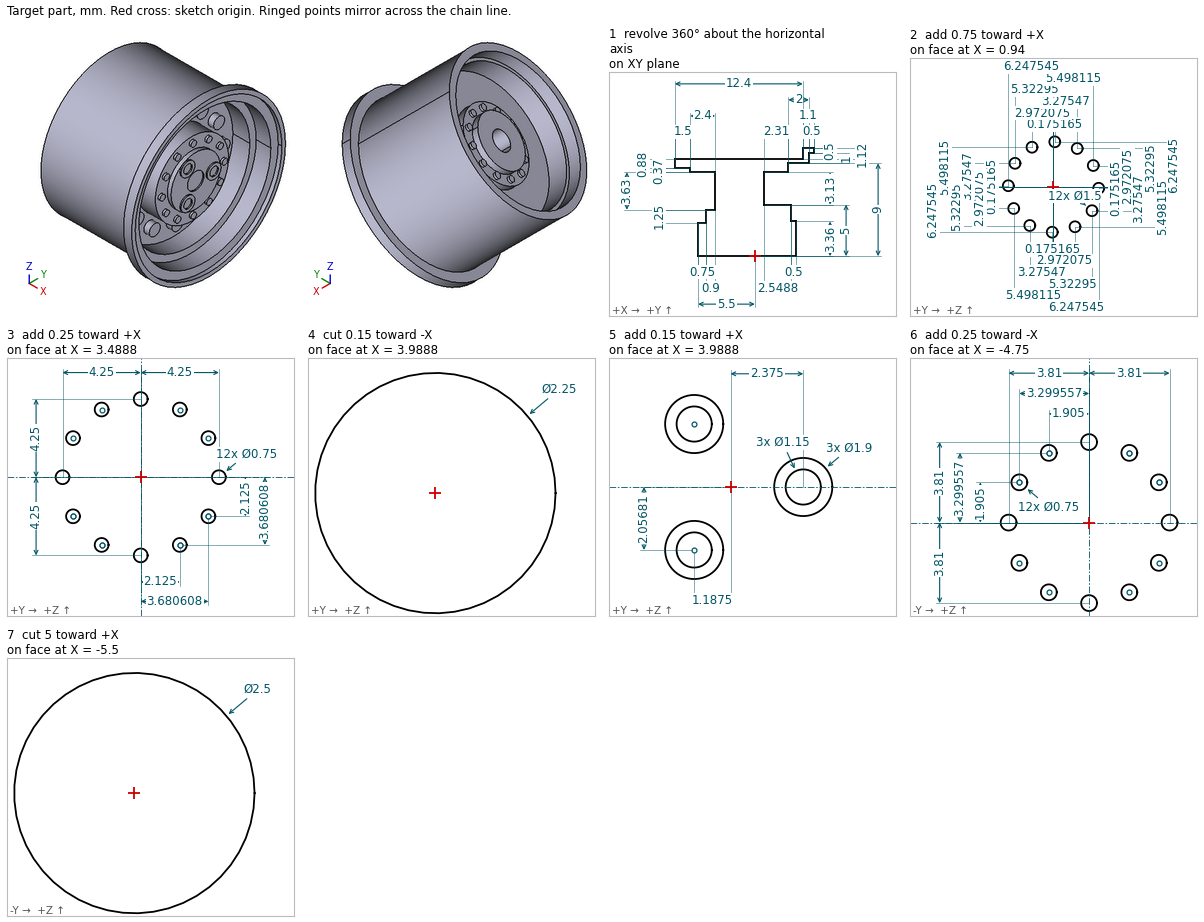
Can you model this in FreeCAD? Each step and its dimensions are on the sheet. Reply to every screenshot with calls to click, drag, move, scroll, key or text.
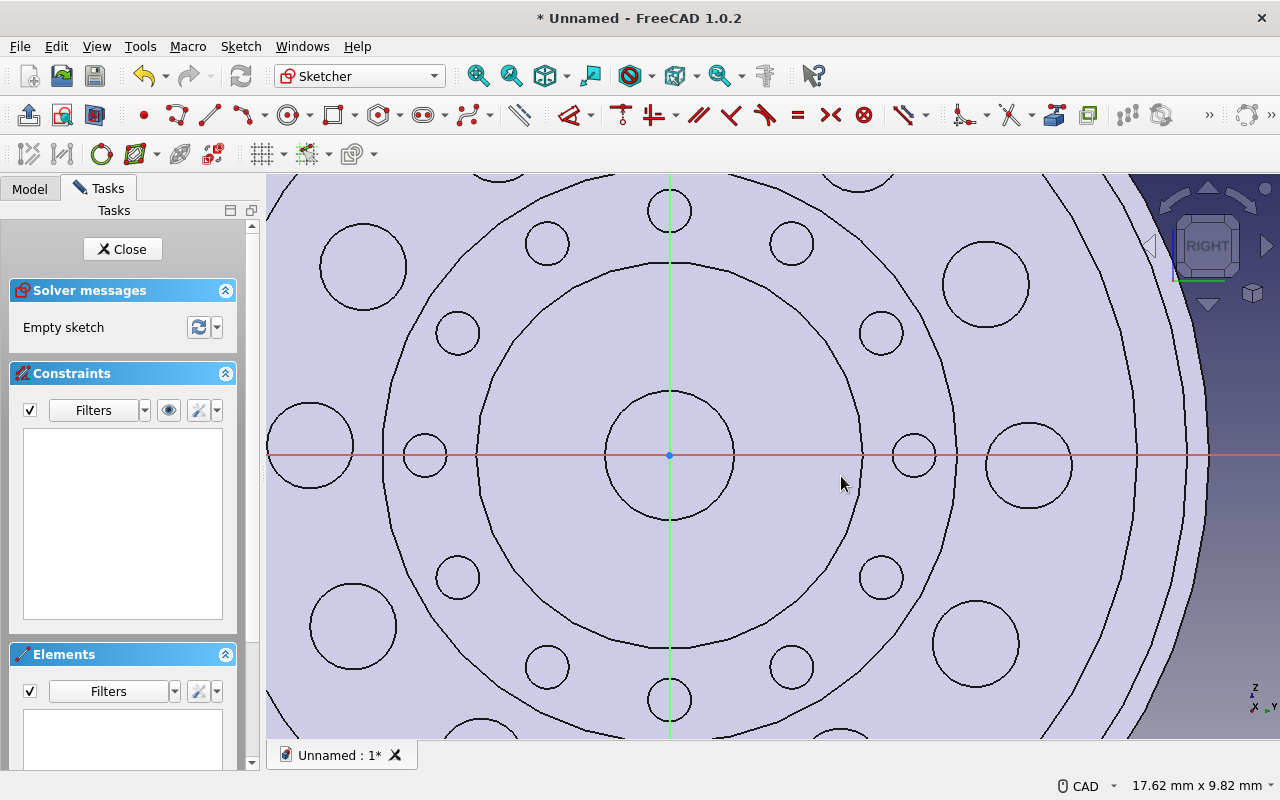
click(288, 116)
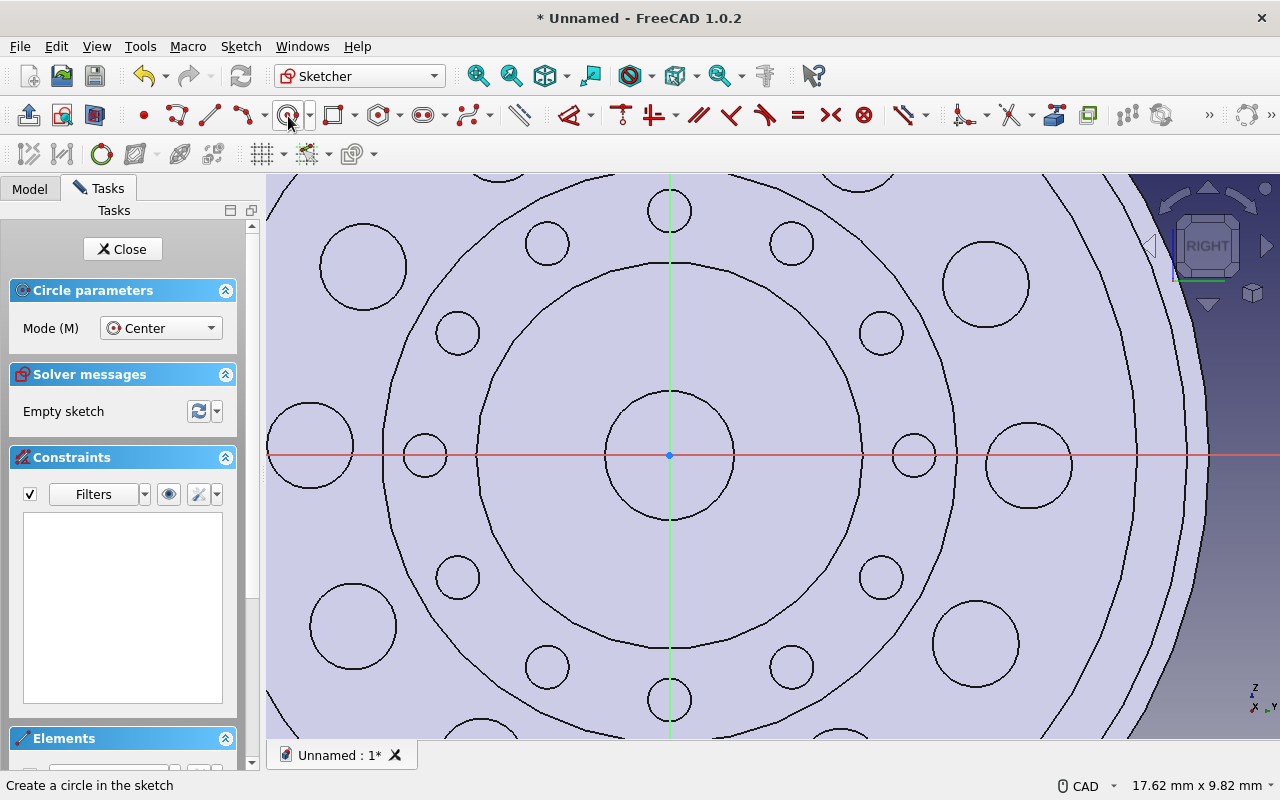
click(806, 455)
move(845, 417)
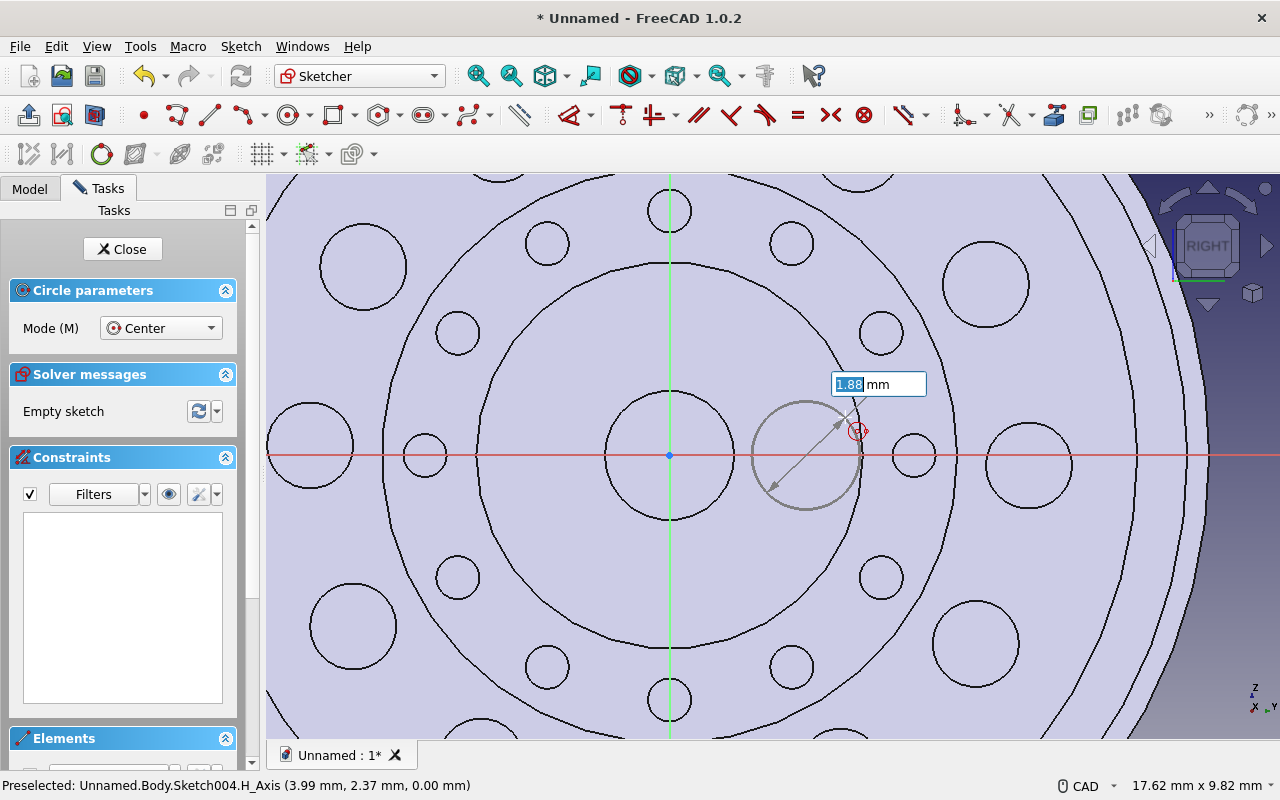
text(1.9)
key(Return)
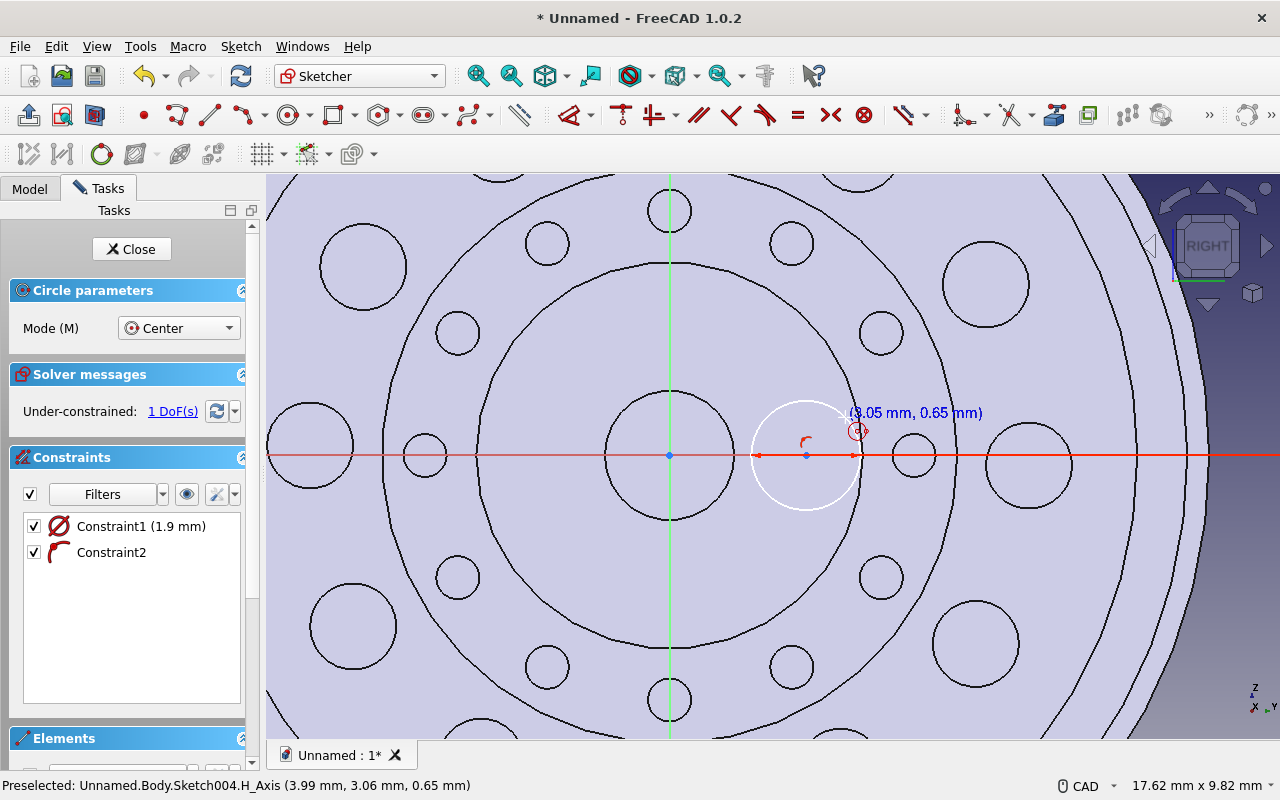
click(601, 574)
move(640, 535)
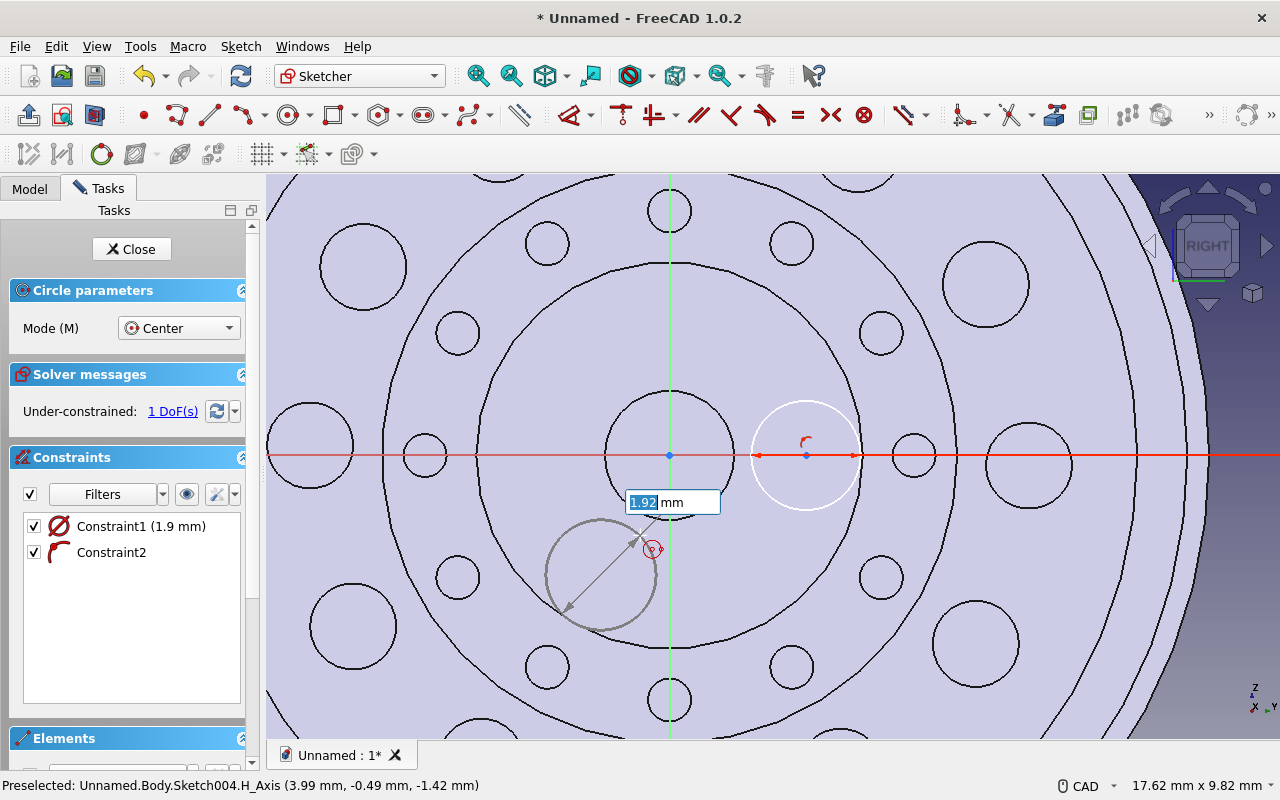
text(1.9)
key(Return)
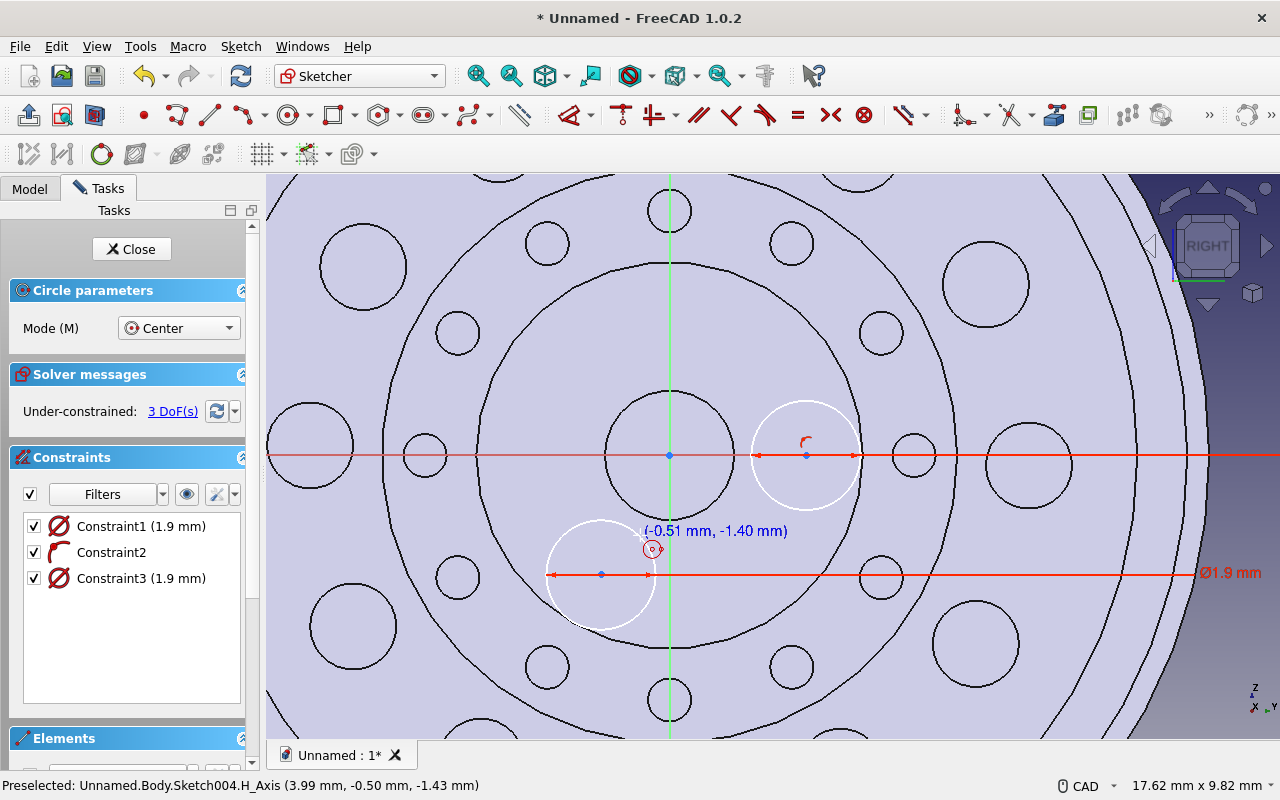
click(601, 337)
move(640, 298)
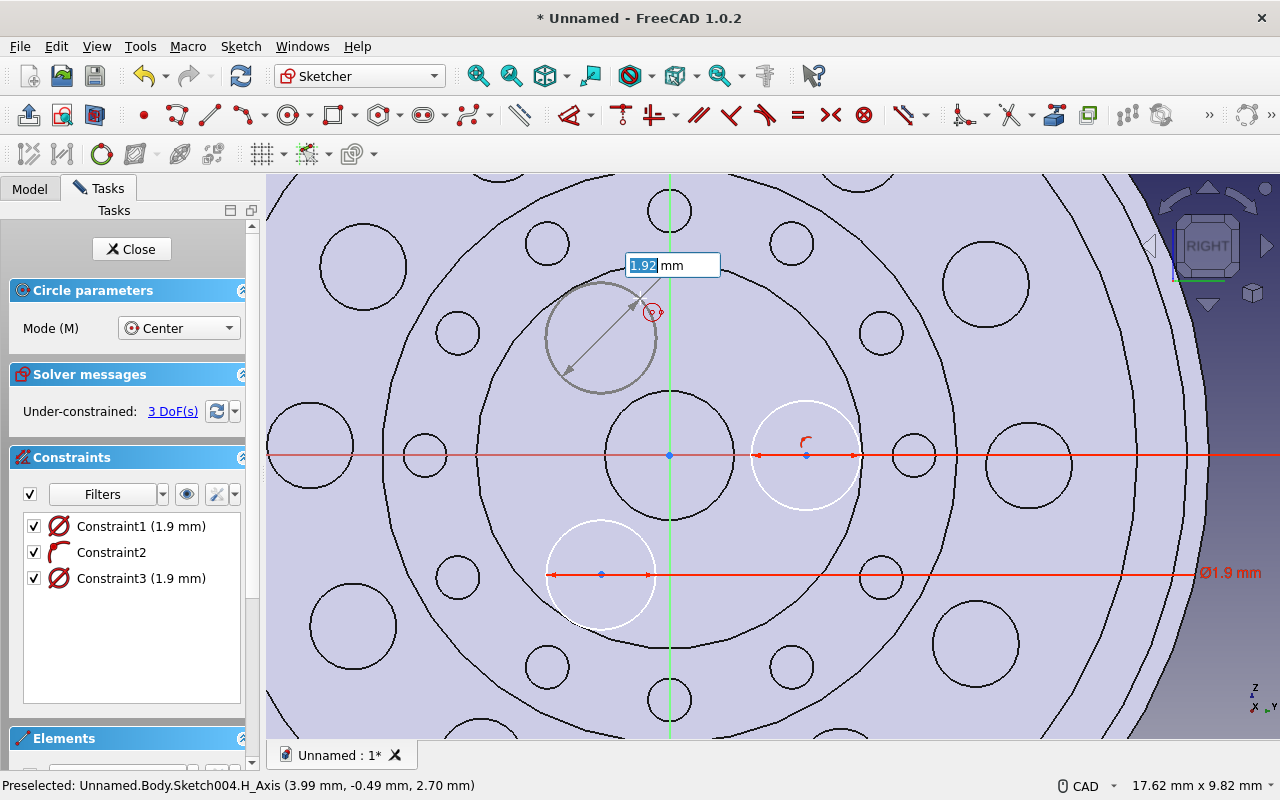
text(1.9)
key(Return)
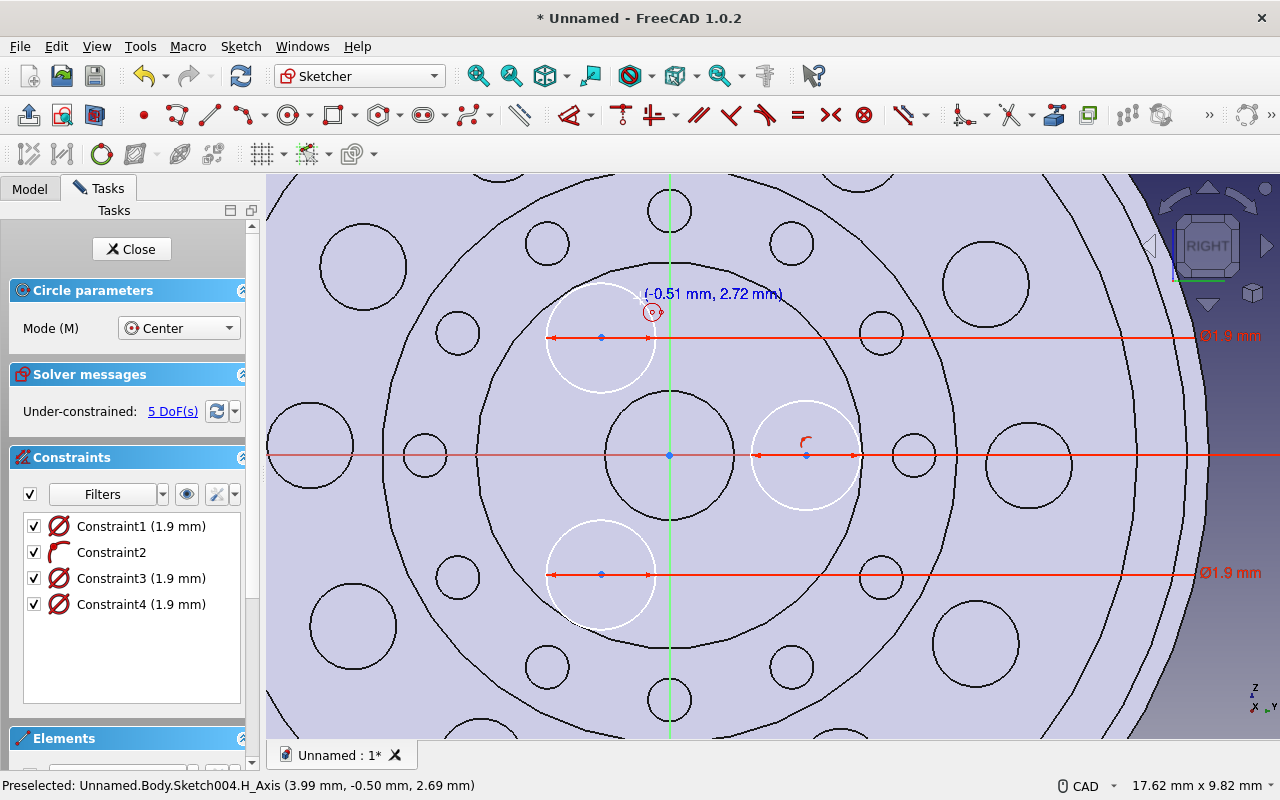
click(806, 455)
move(830, 432)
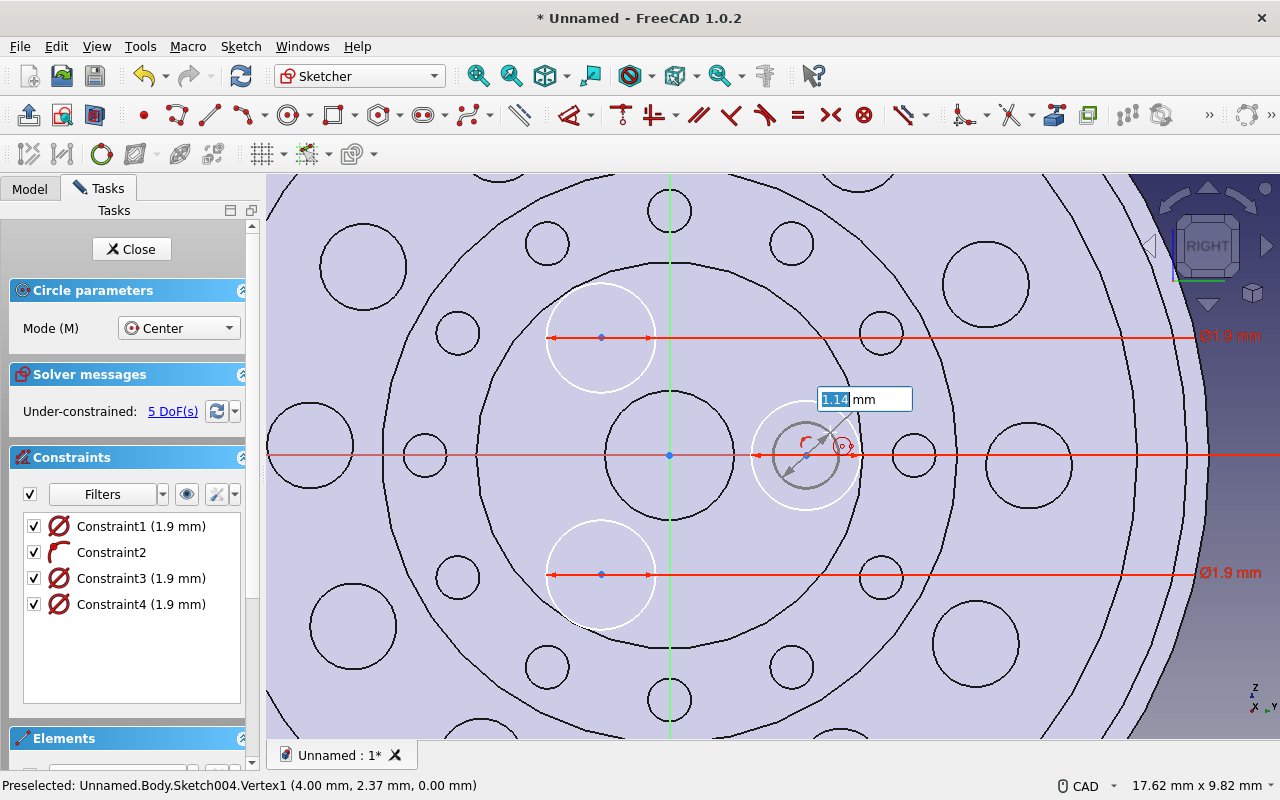
text(1.15)
key(Return)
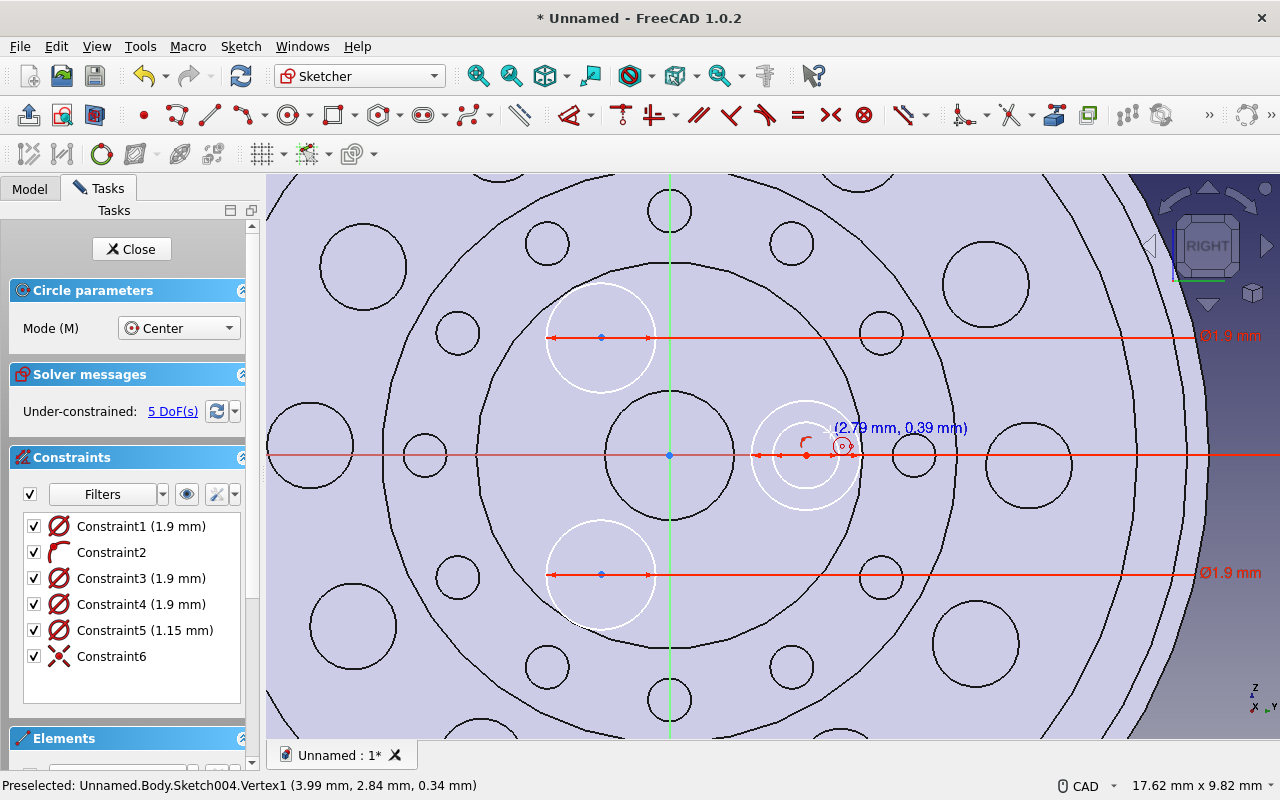
click(601, 575)
move(625, 550)